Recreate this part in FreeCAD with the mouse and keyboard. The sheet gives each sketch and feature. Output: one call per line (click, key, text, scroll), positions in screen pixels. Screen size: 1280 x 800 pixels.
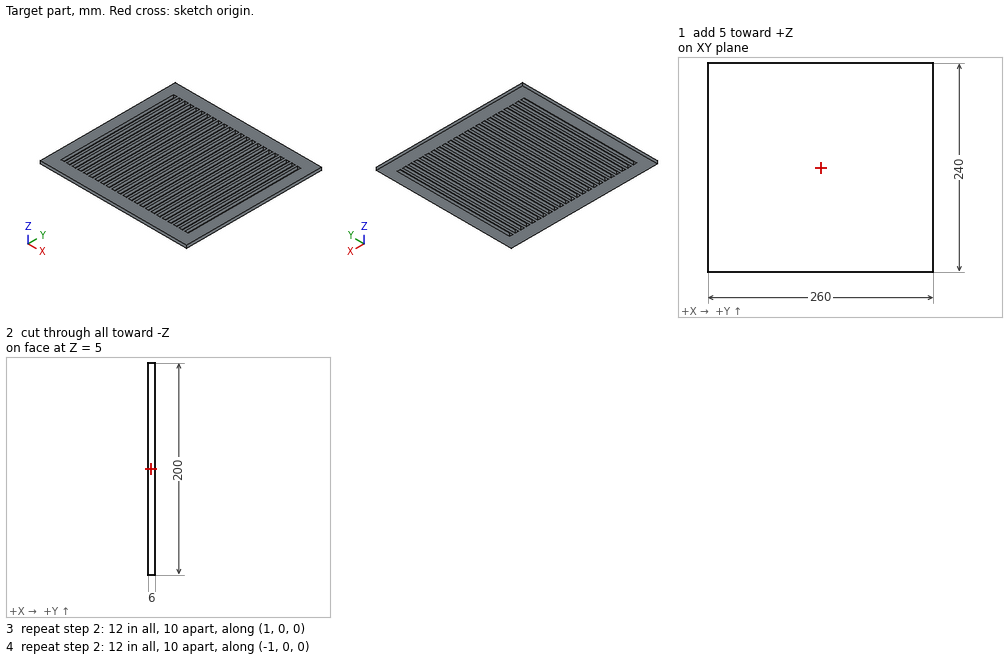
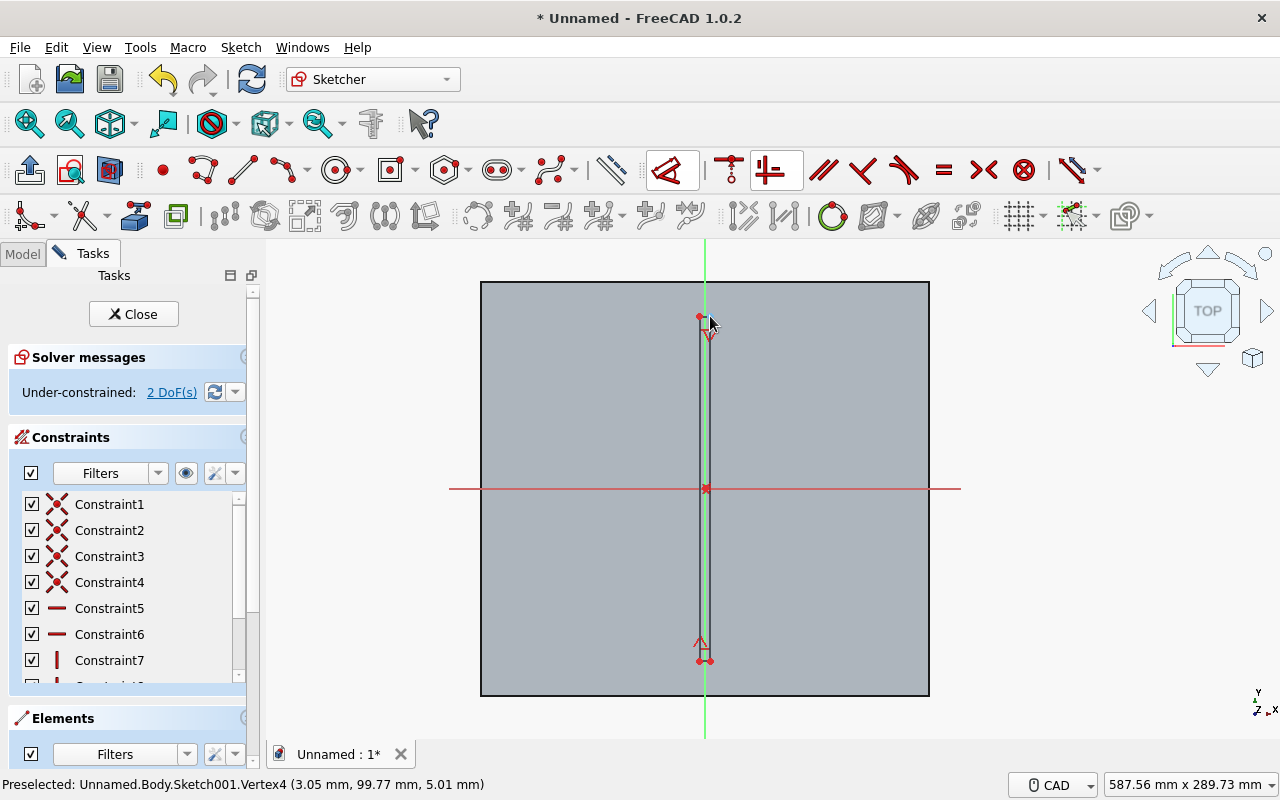
scroll(704, 661, up, 7)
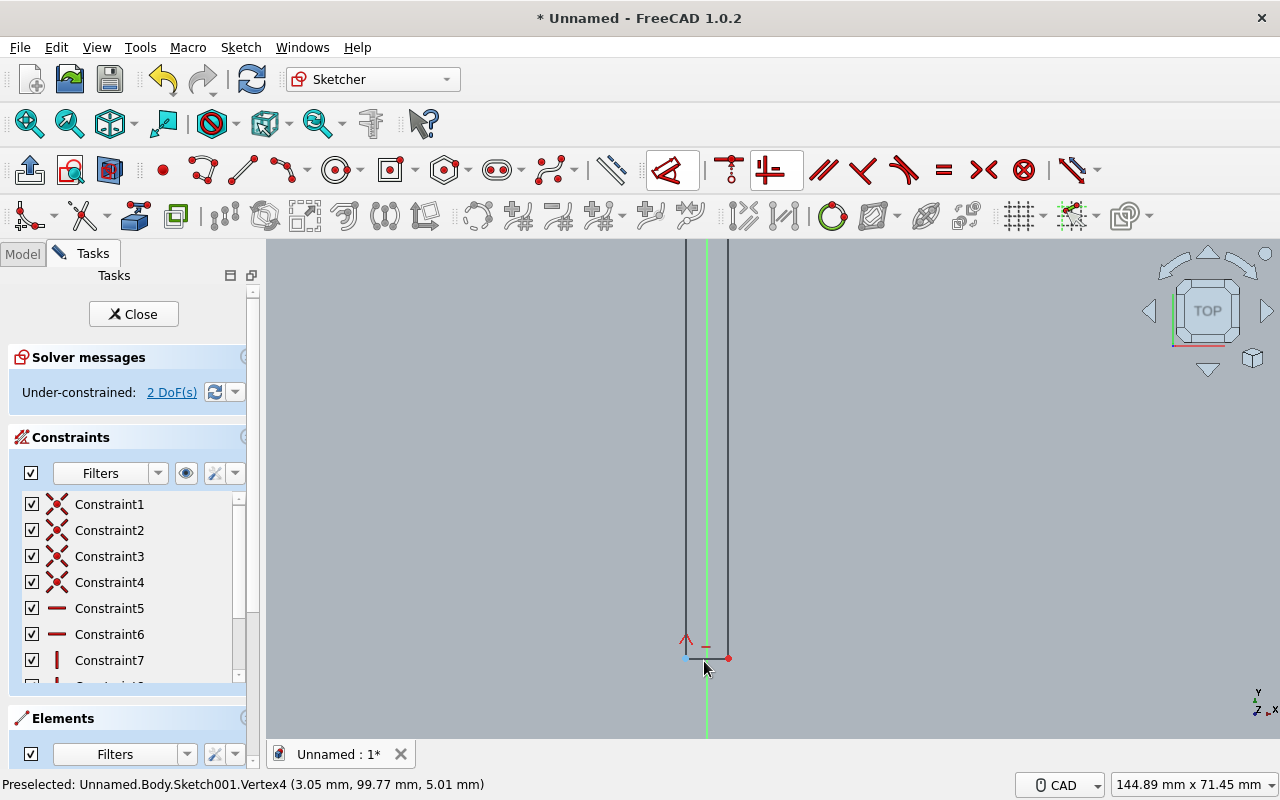
click(703, 659)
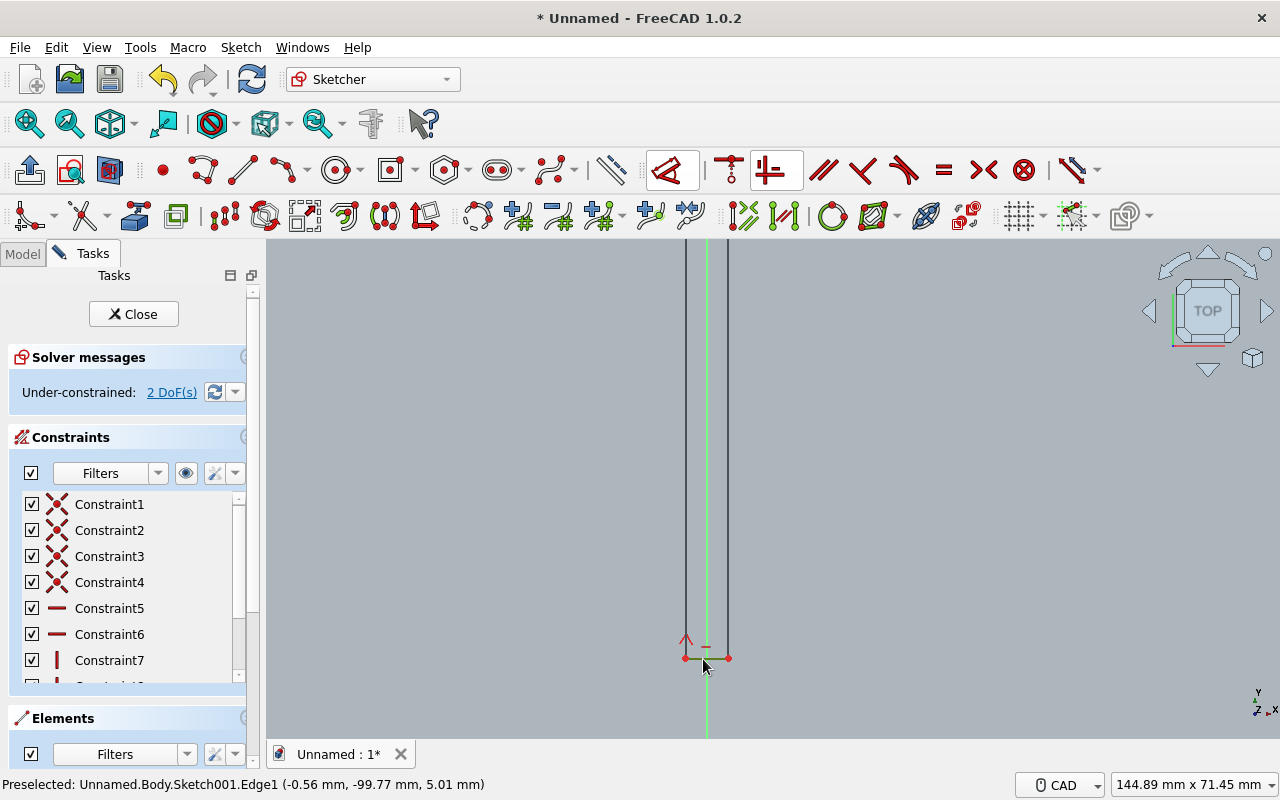
key(l)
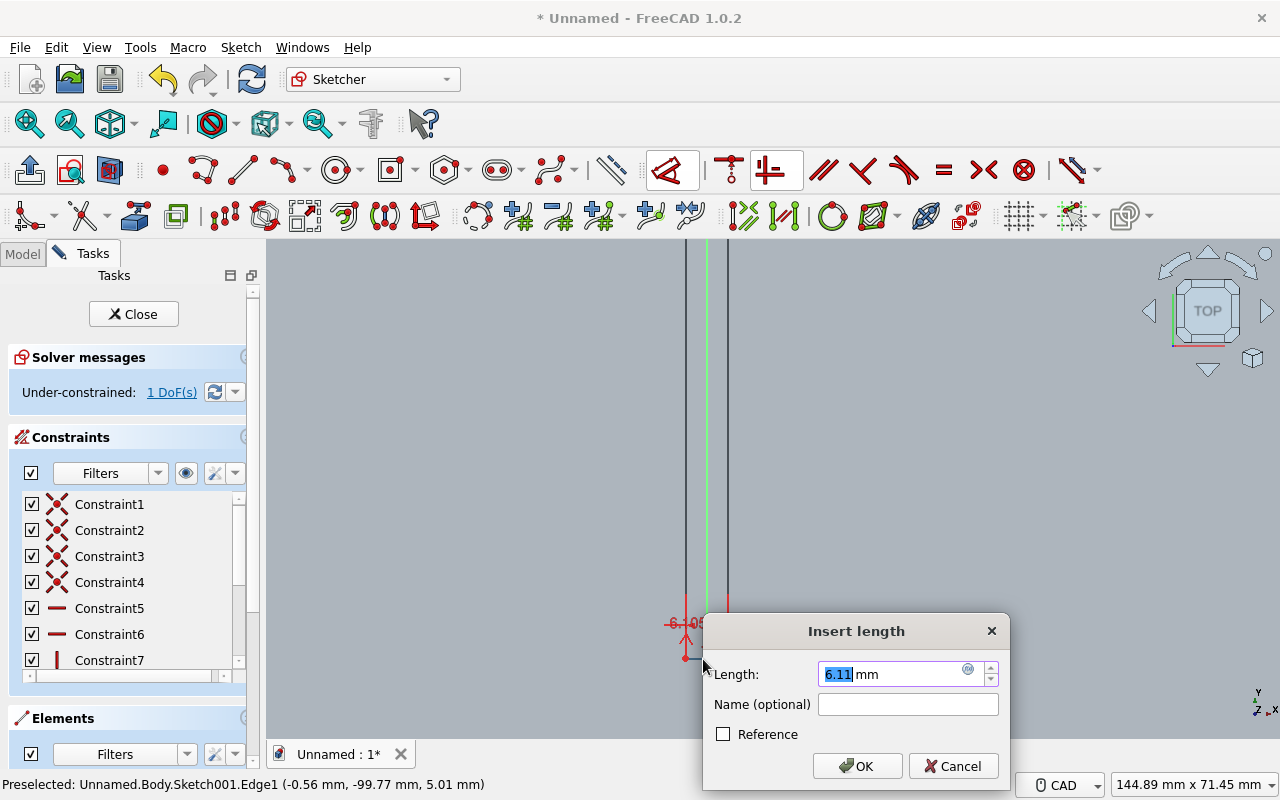
text(6)
key(Return)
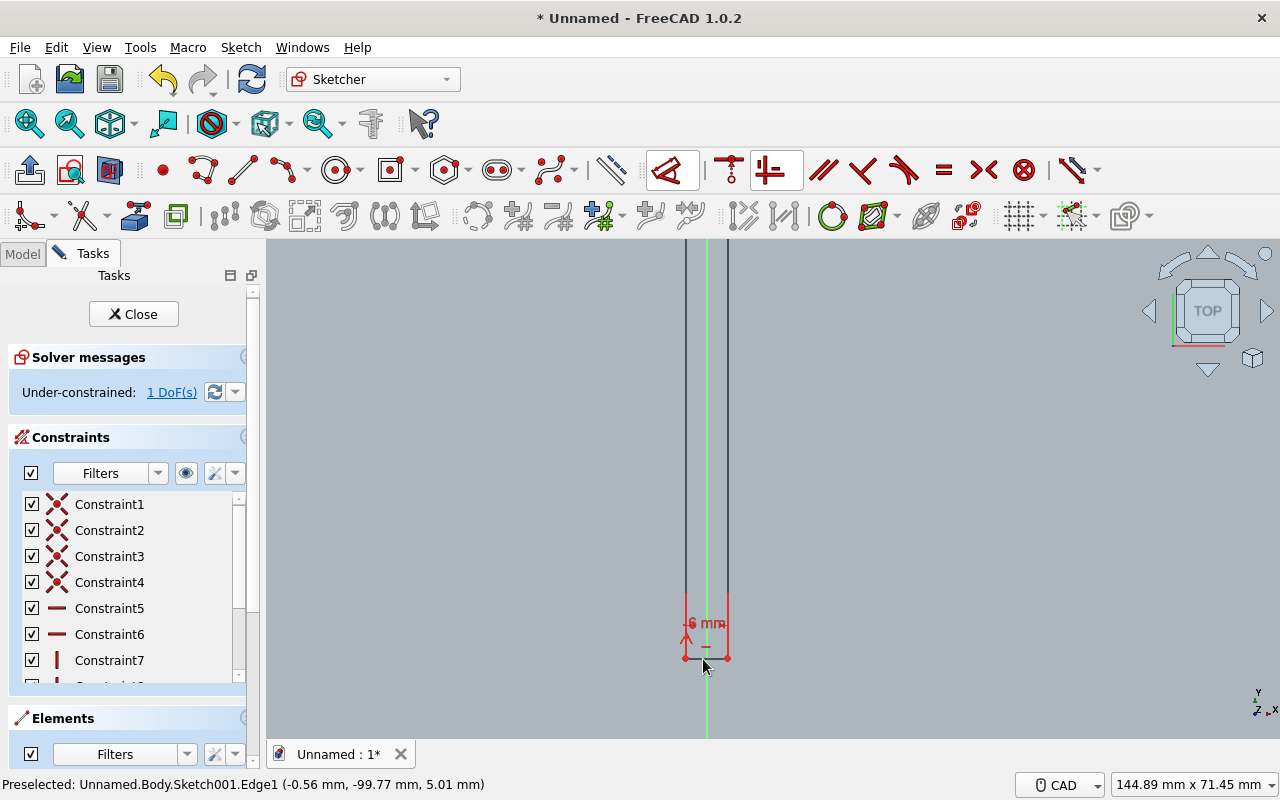
click(728, 379)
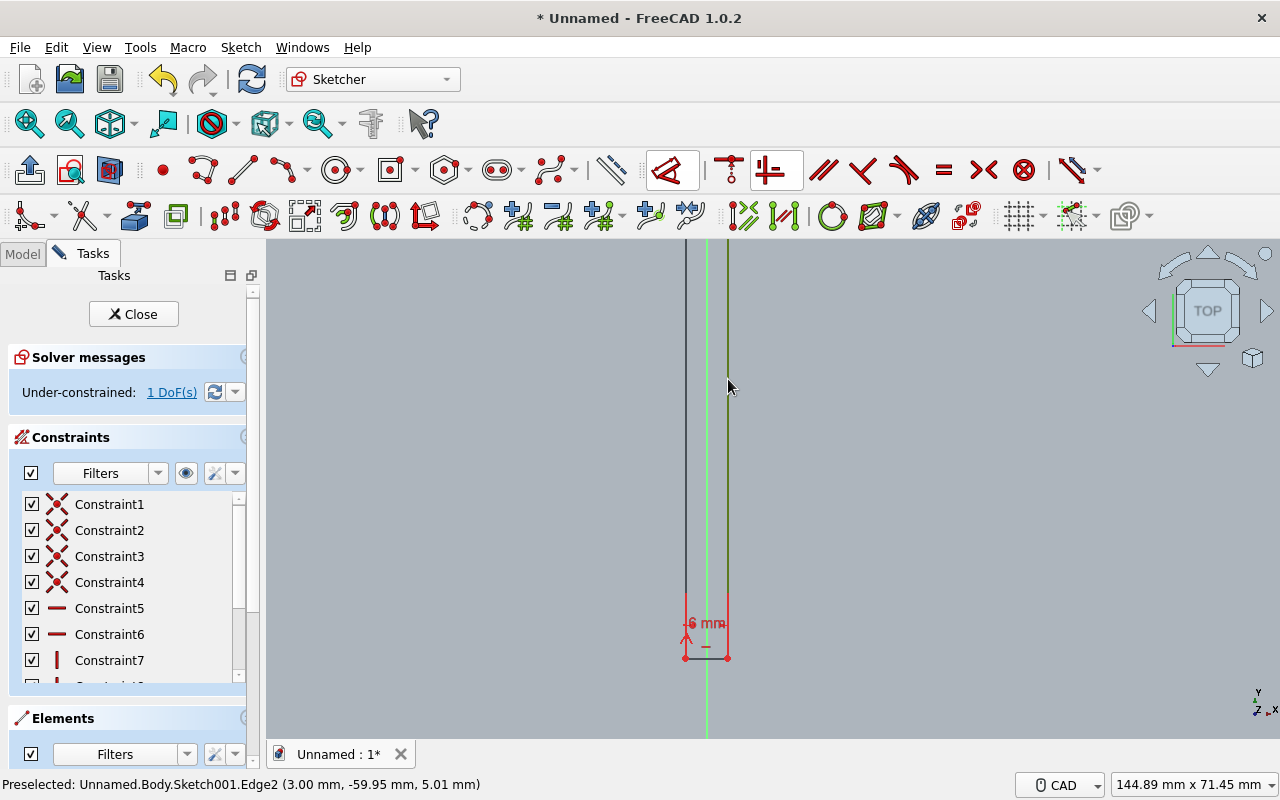
key(i)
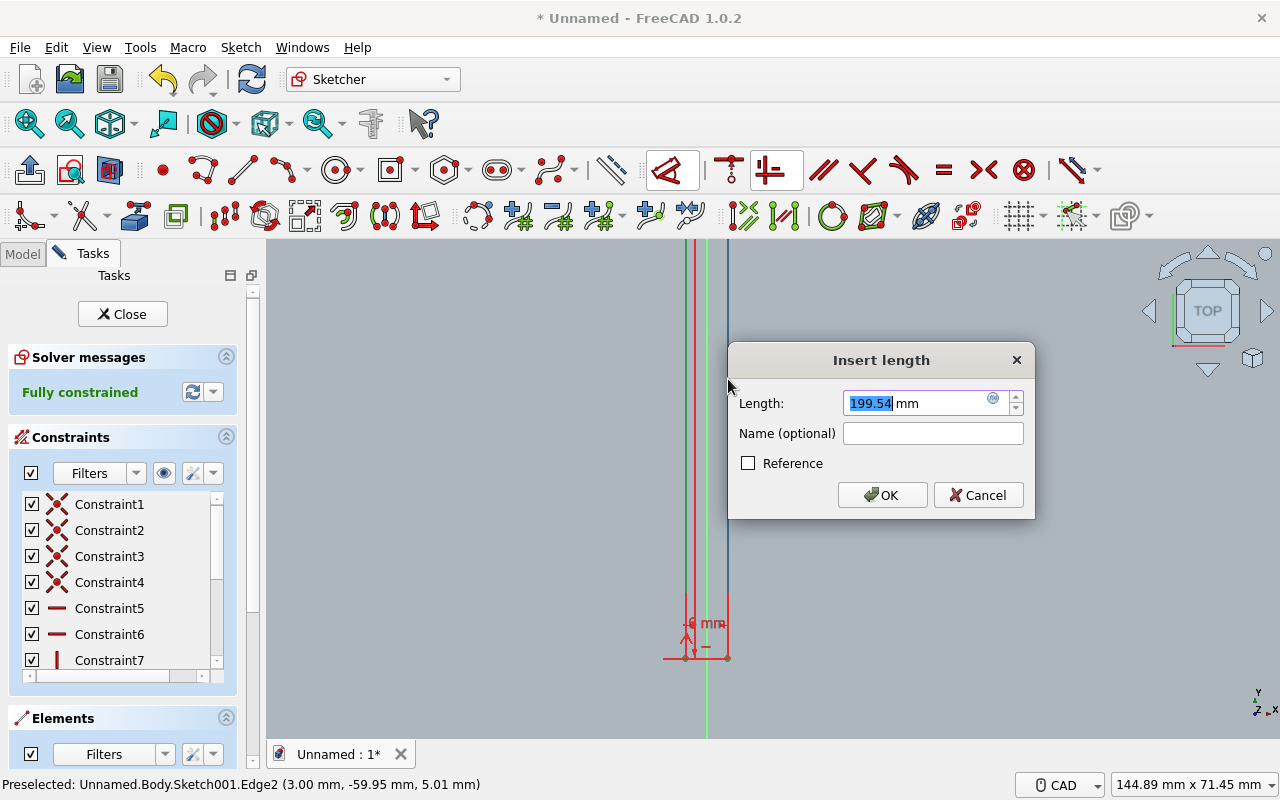
text(200)
key(Return)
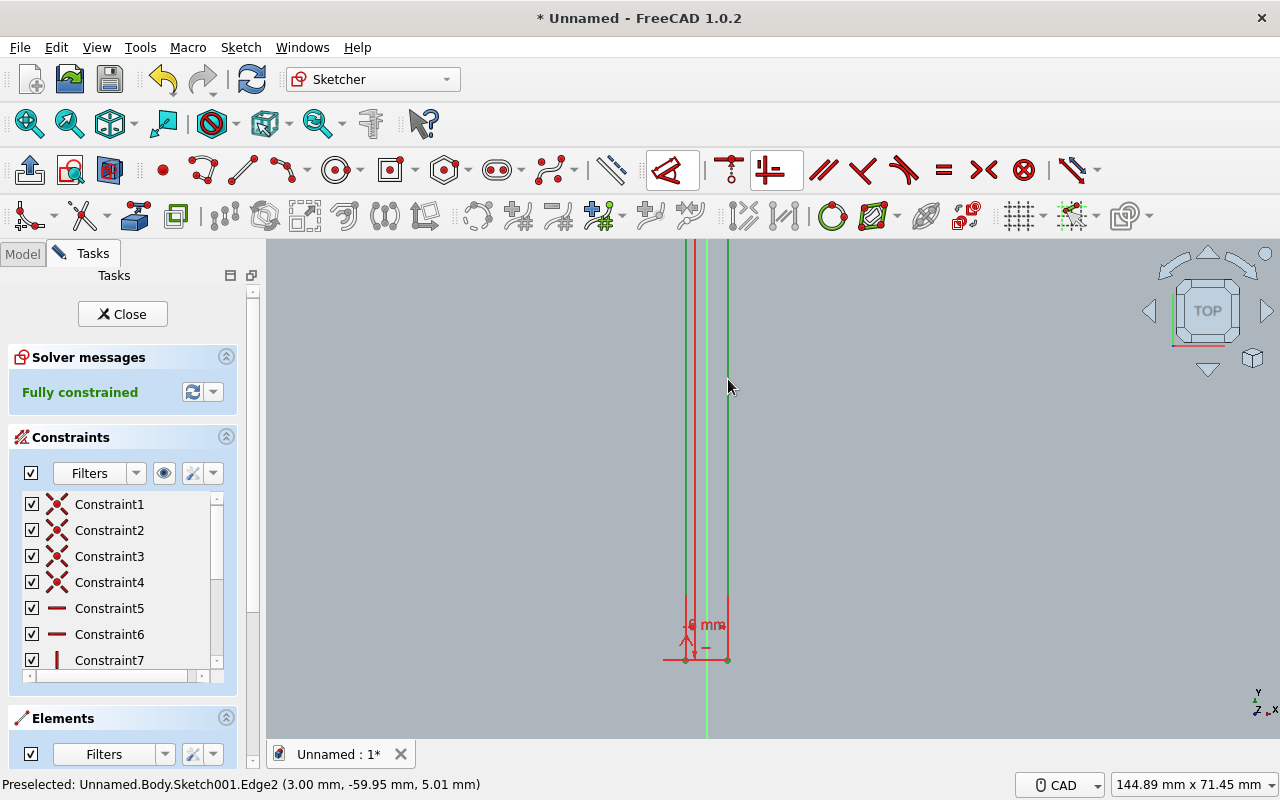
click(123, 314)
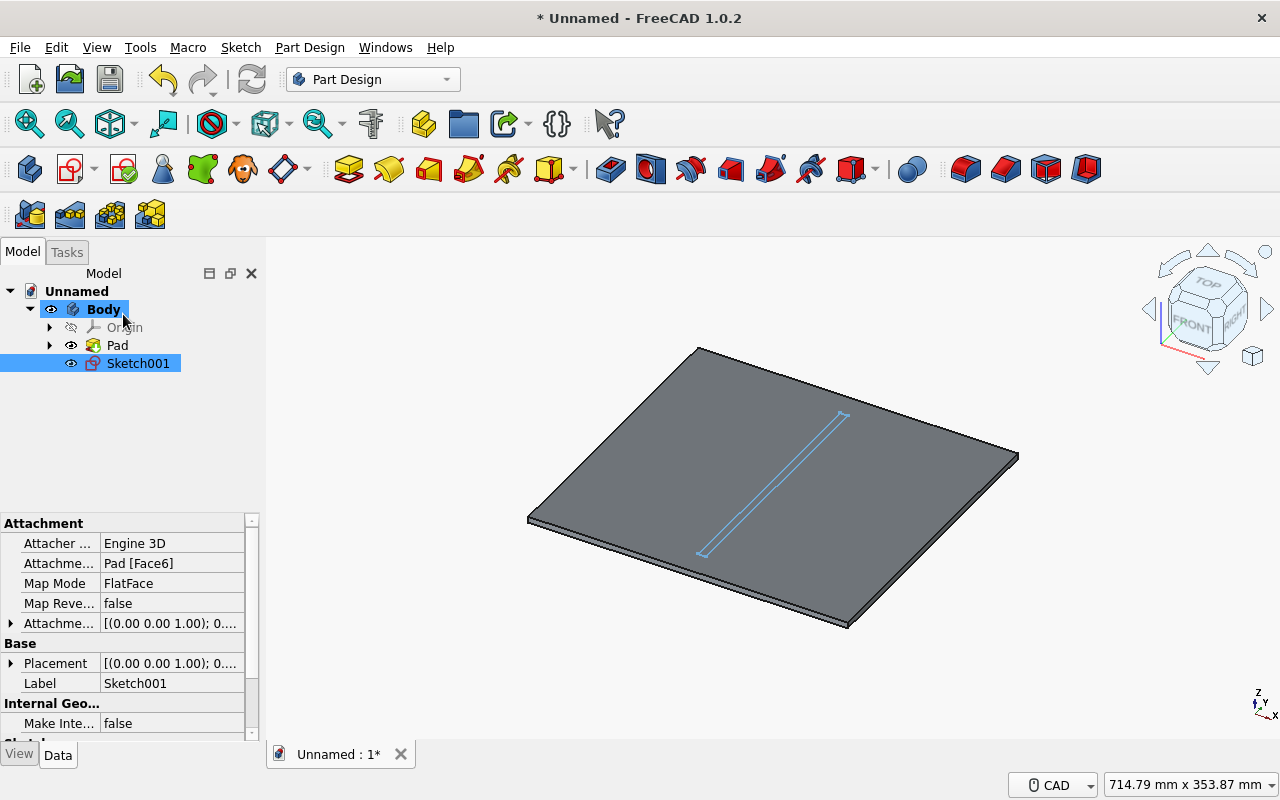
click(612, 170)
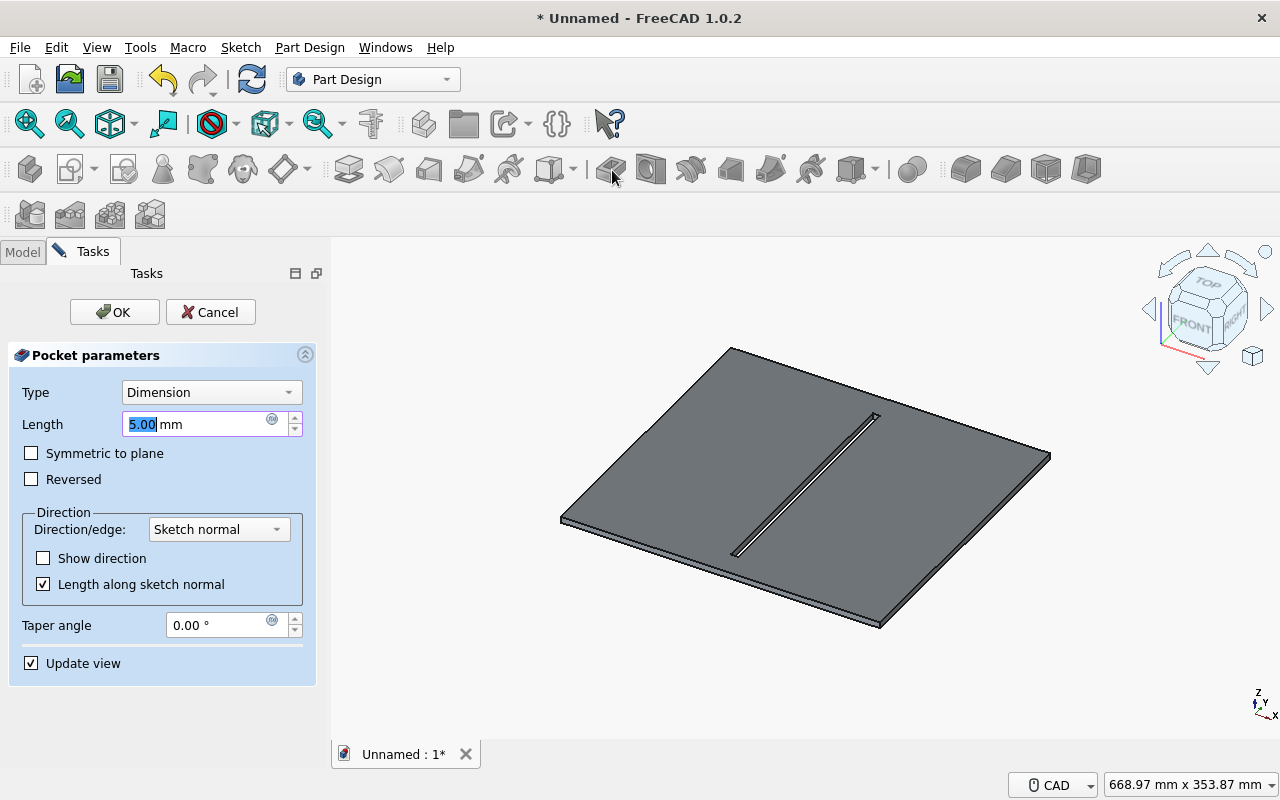
click(212, 392)